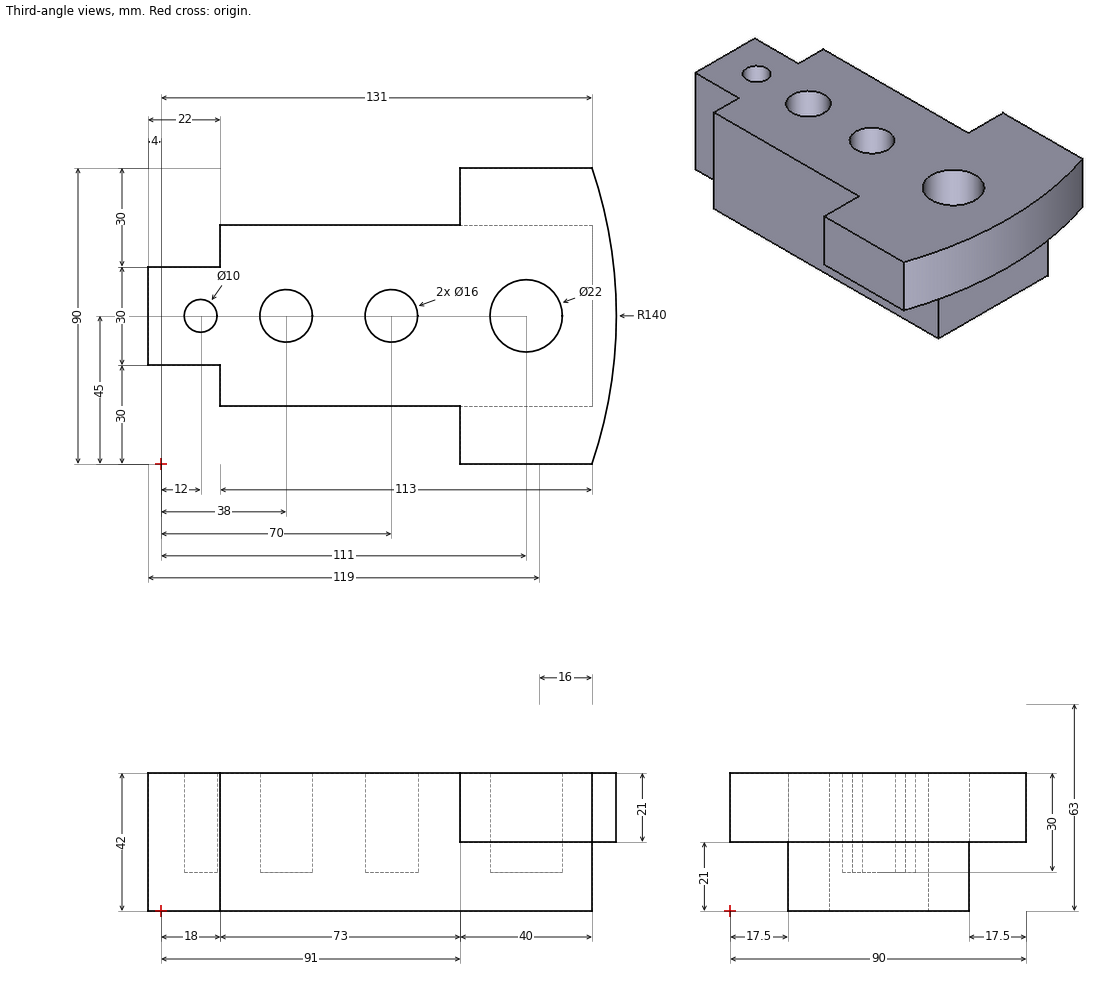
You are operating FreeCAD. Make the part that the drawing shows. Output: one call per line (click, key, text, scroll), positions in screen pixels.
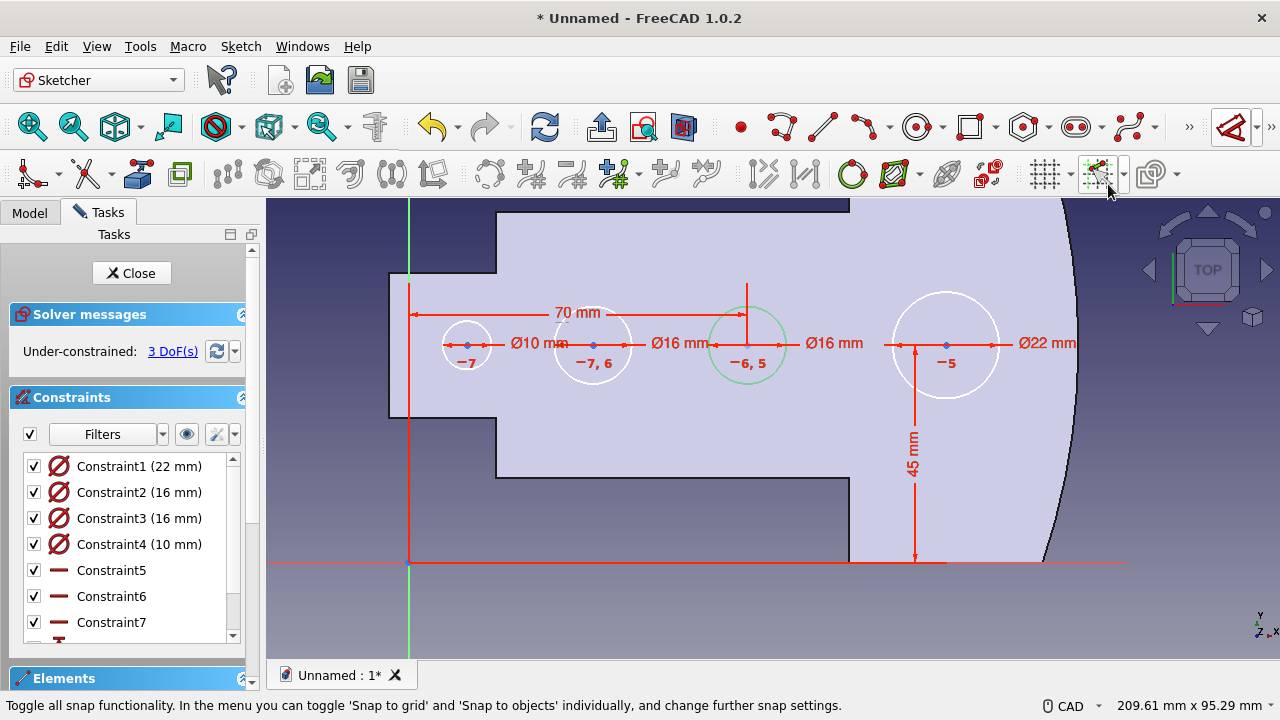
click(593, 345)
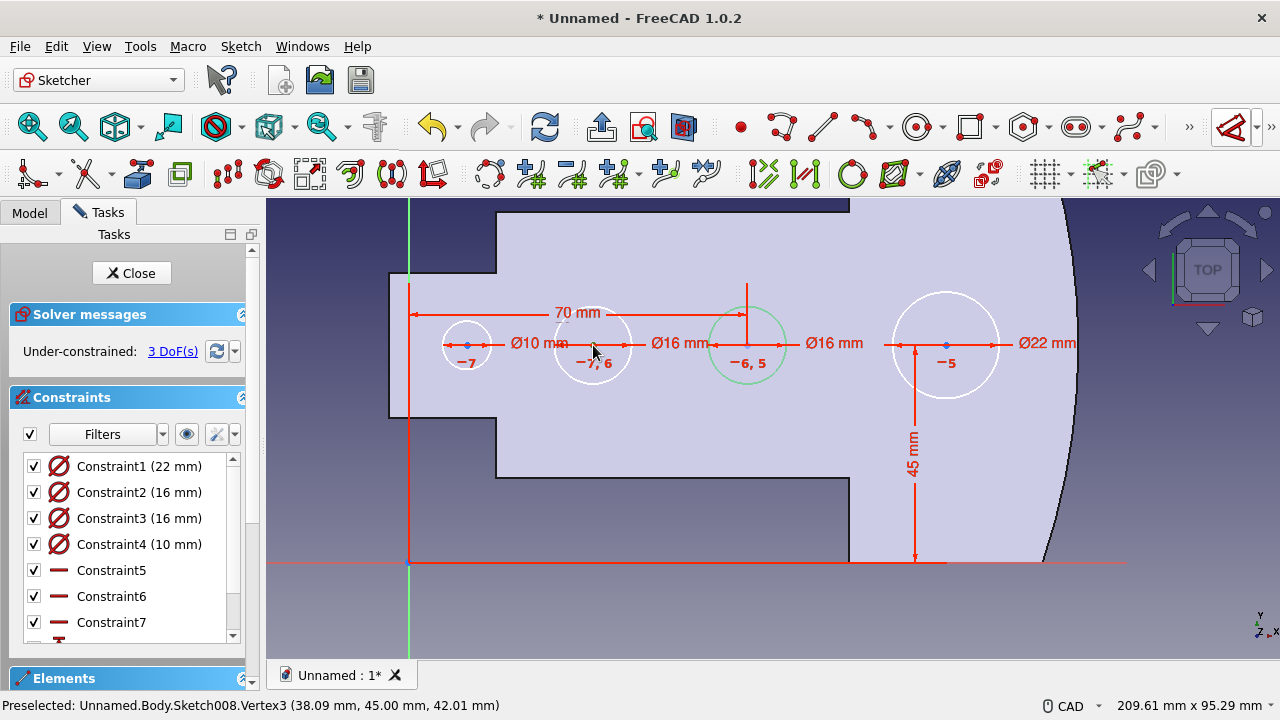
key(l)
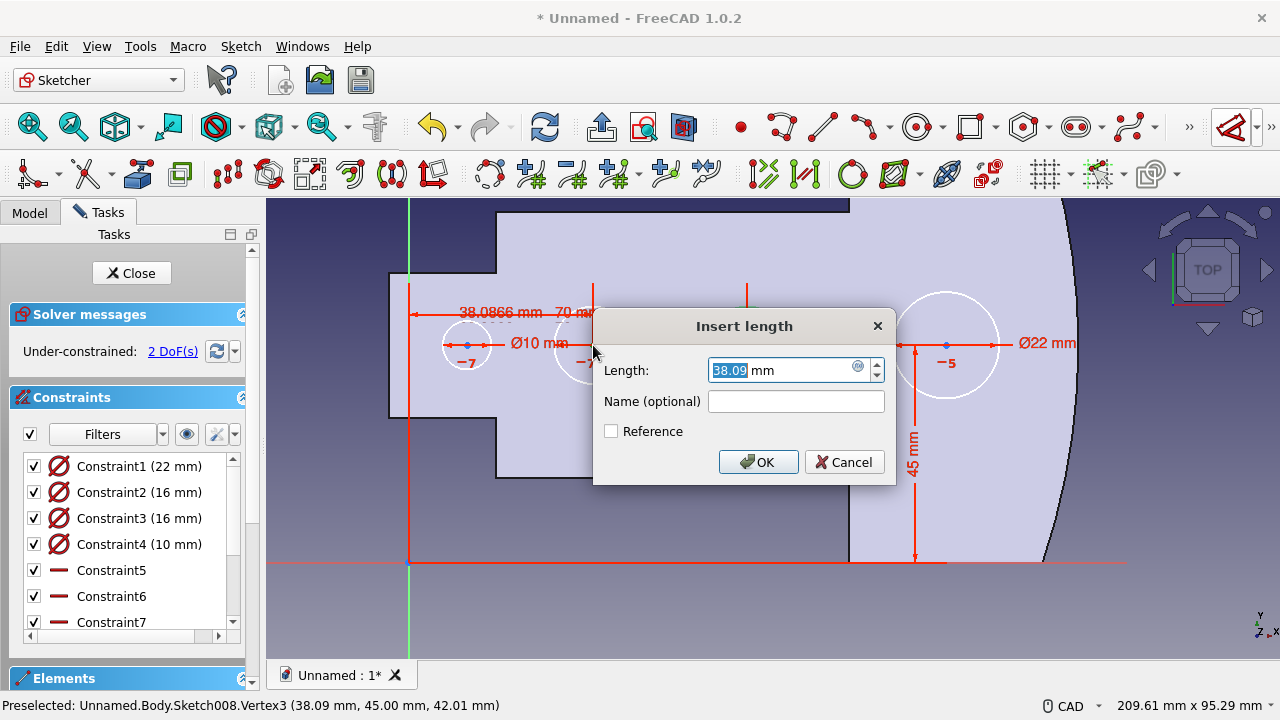
text(38)
key(Return)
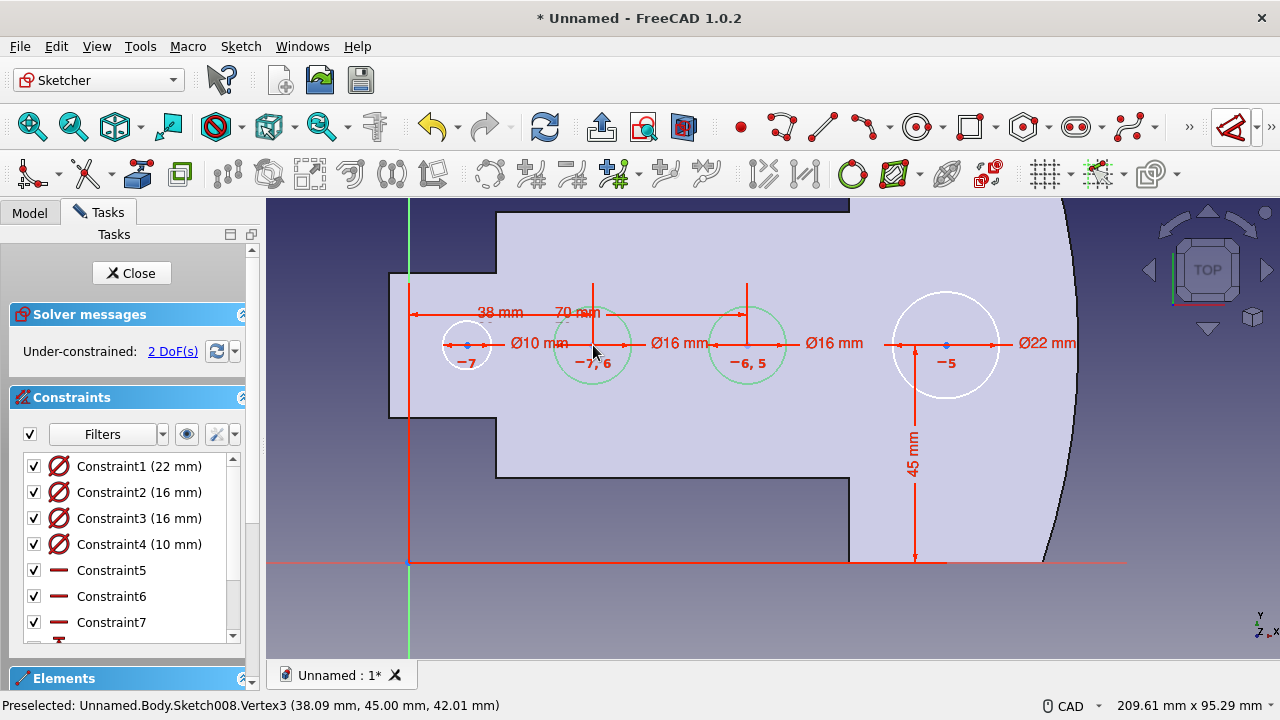
click(467, 345)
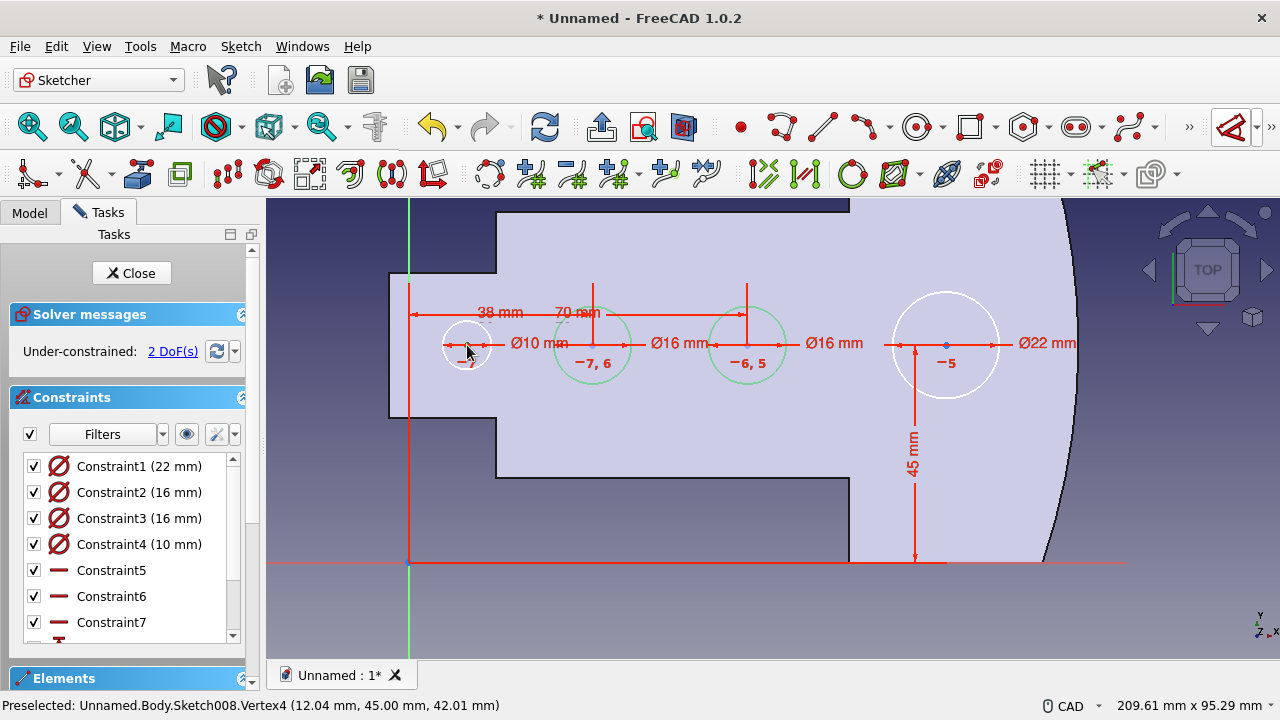
click(1256, 128)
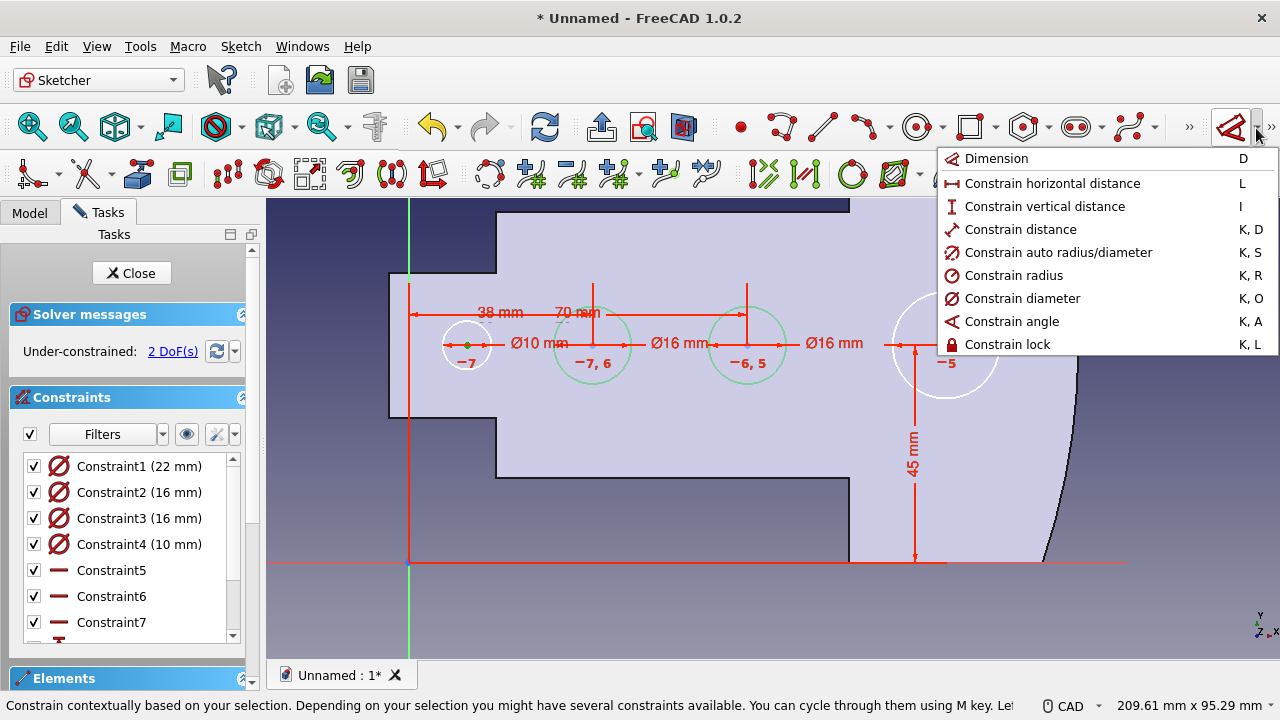
click(1108, 184)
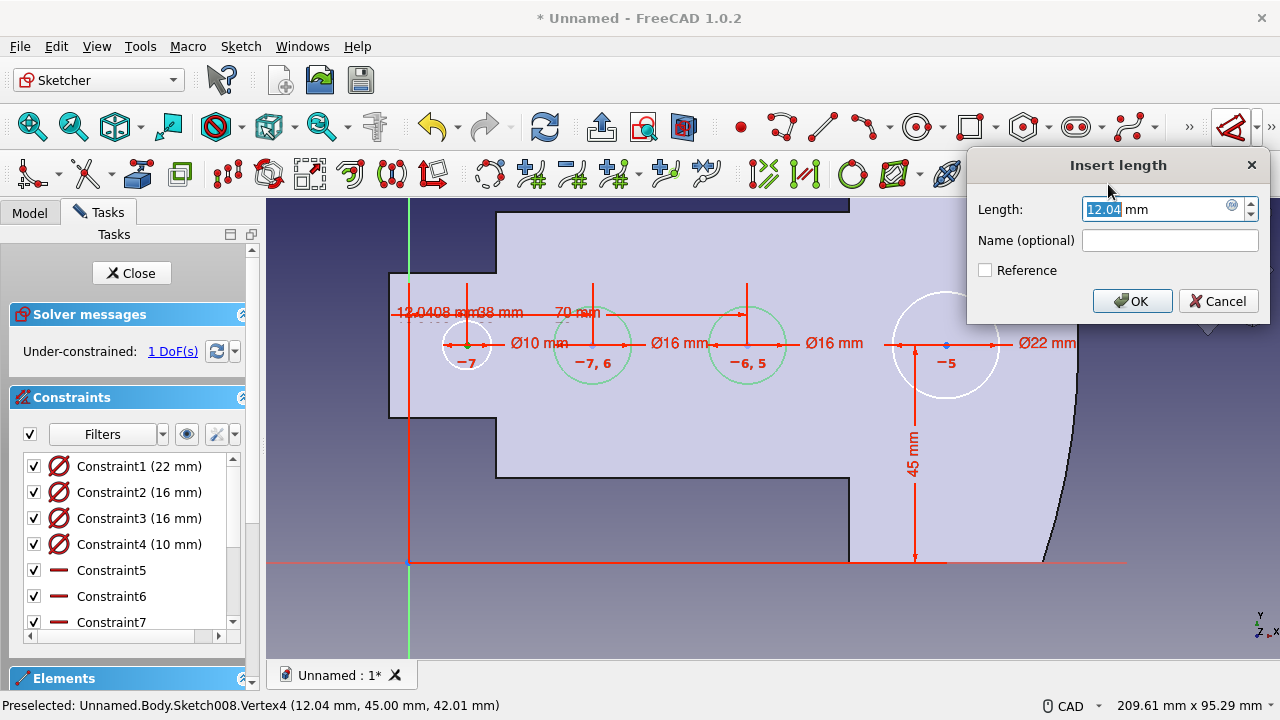
text(12)
key(Return)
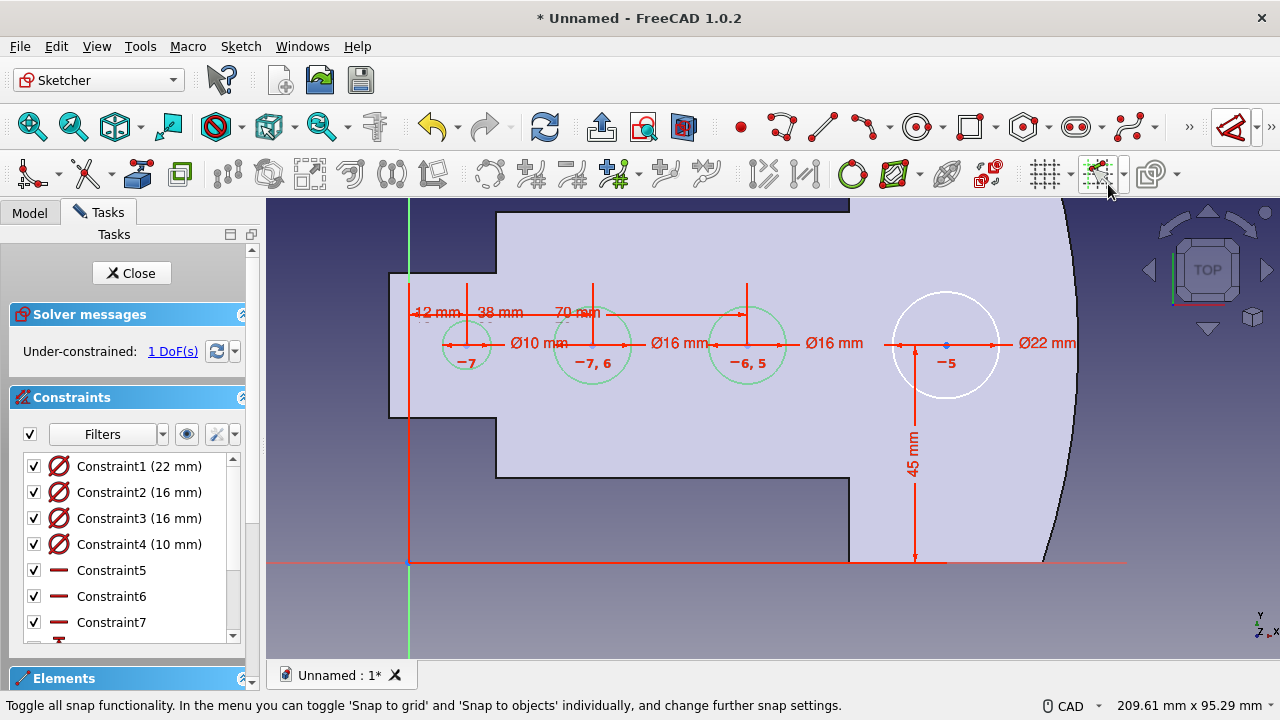
click(946, 345)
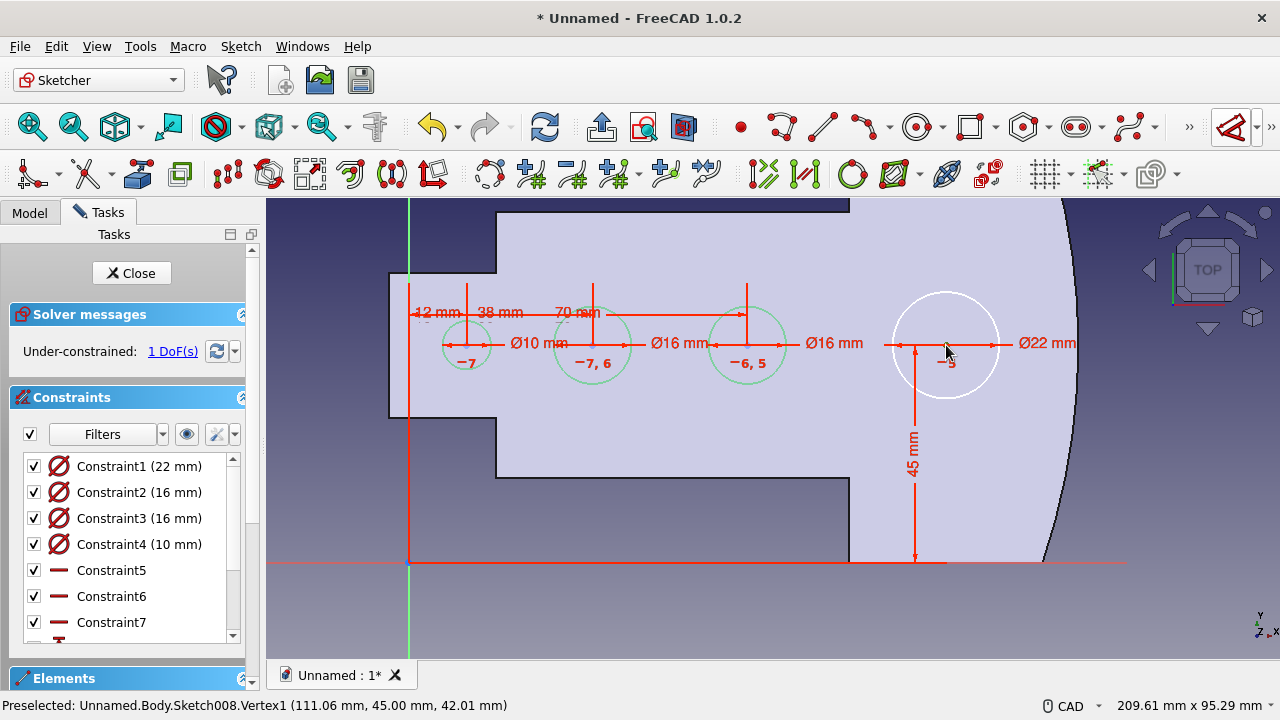
key(l)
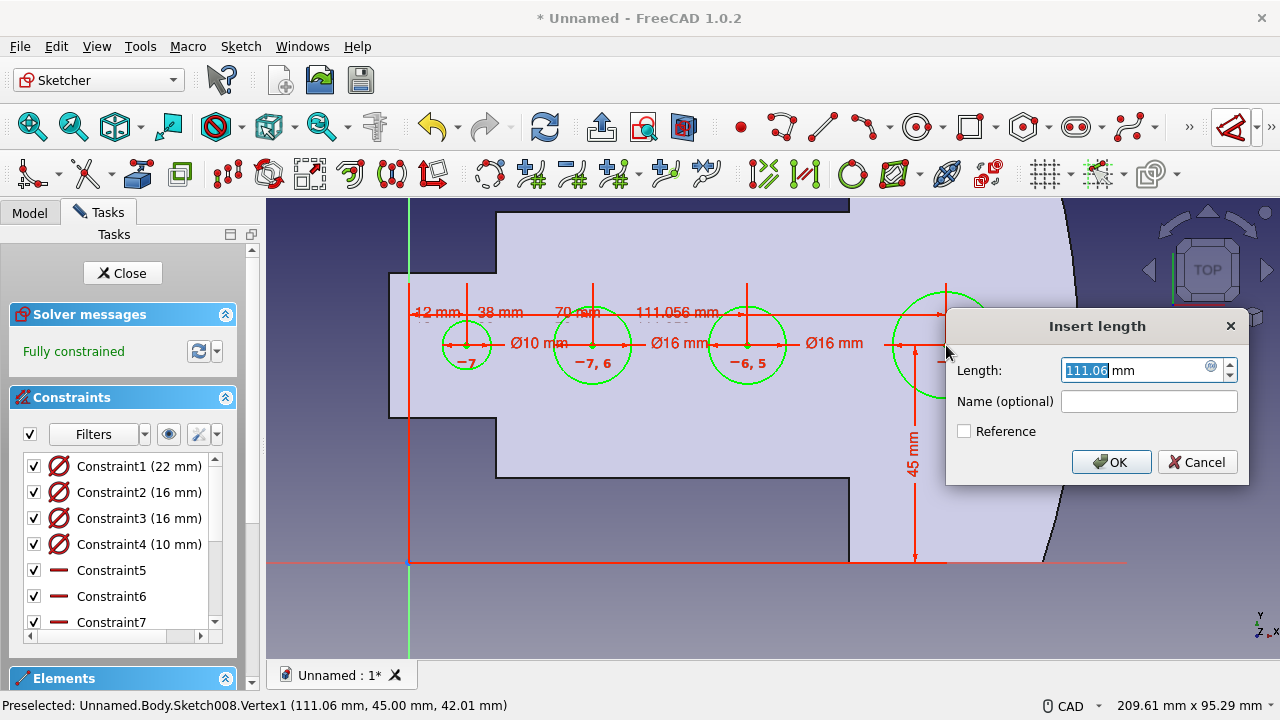
text(111)
key(Return)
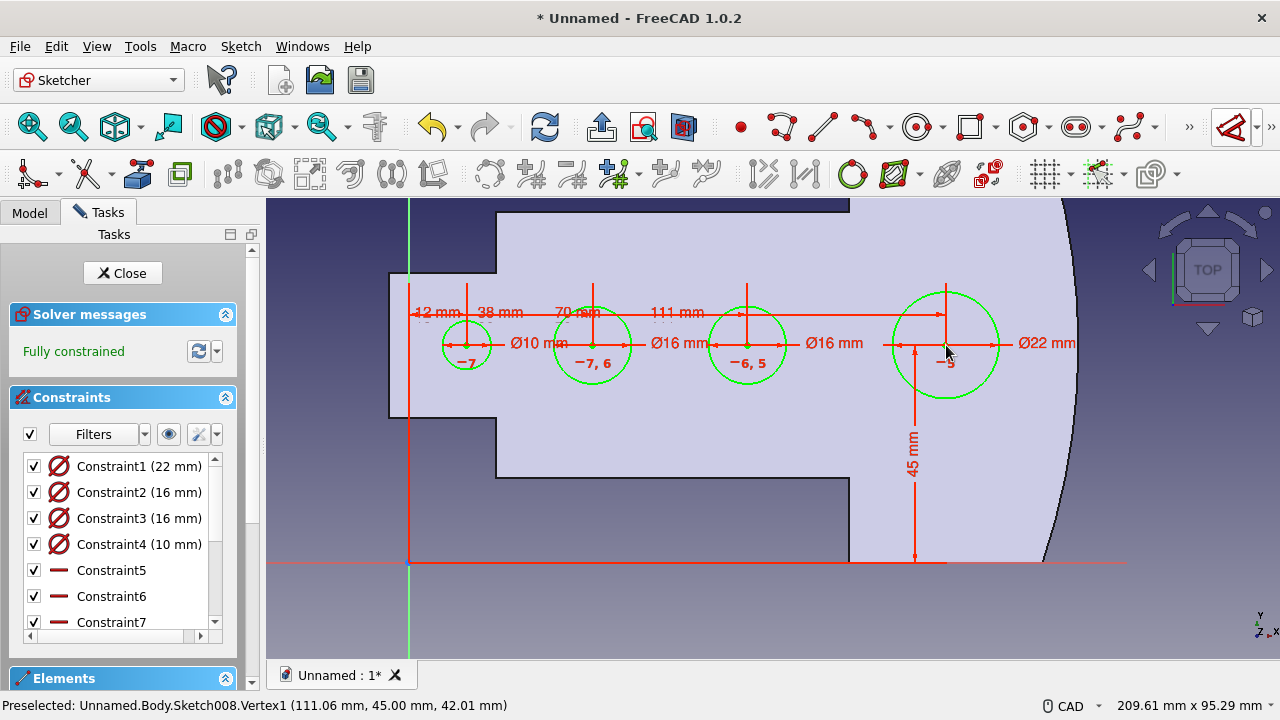
click(123, 273)